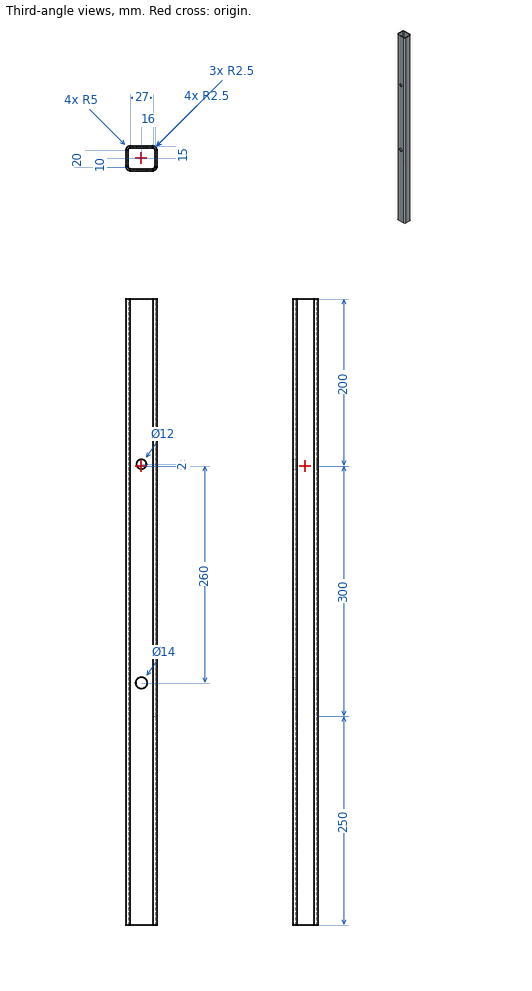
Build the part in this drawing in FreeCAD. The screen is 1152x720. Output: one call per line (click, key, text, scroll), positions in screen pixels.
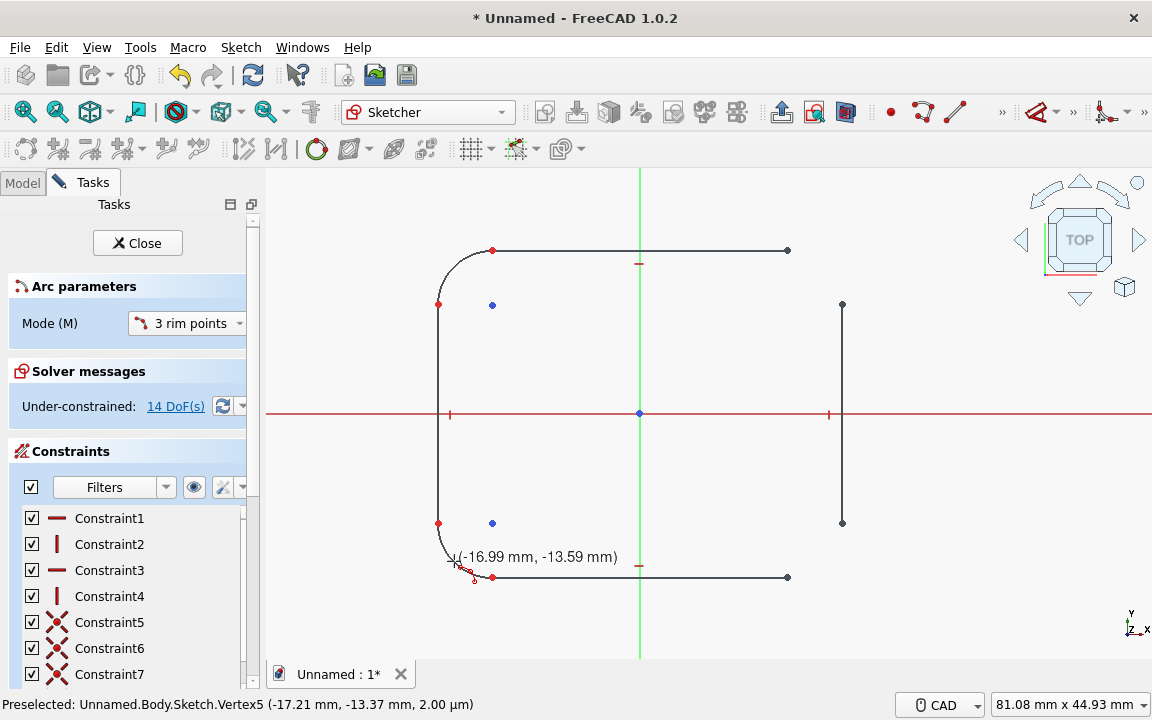
click(787, 578)
click(842, 524)
click(826, 561)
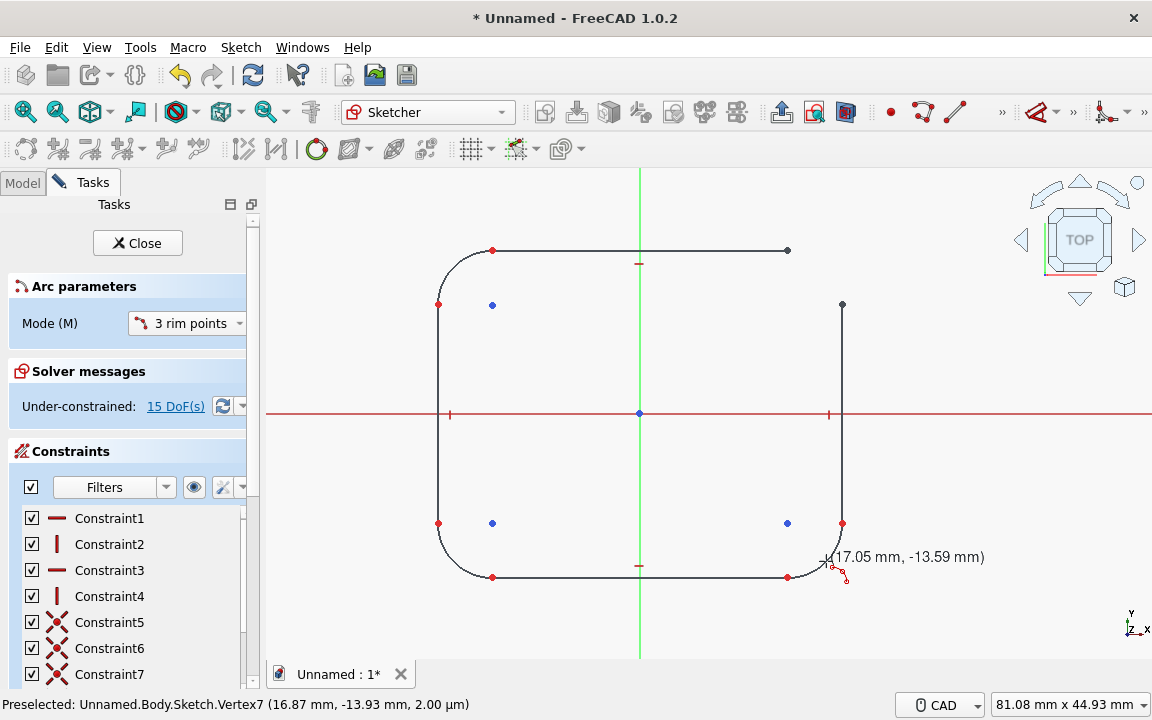
click(842, 305)
click(787, 251)
click(826, 266)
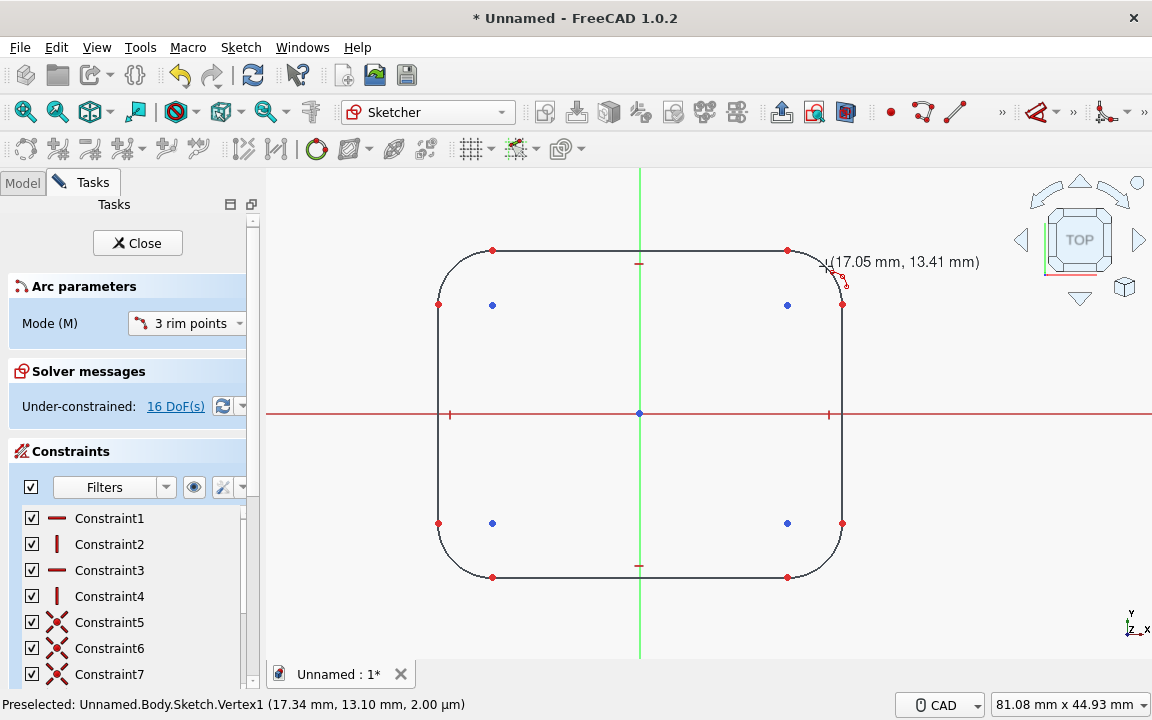
click(956, 112)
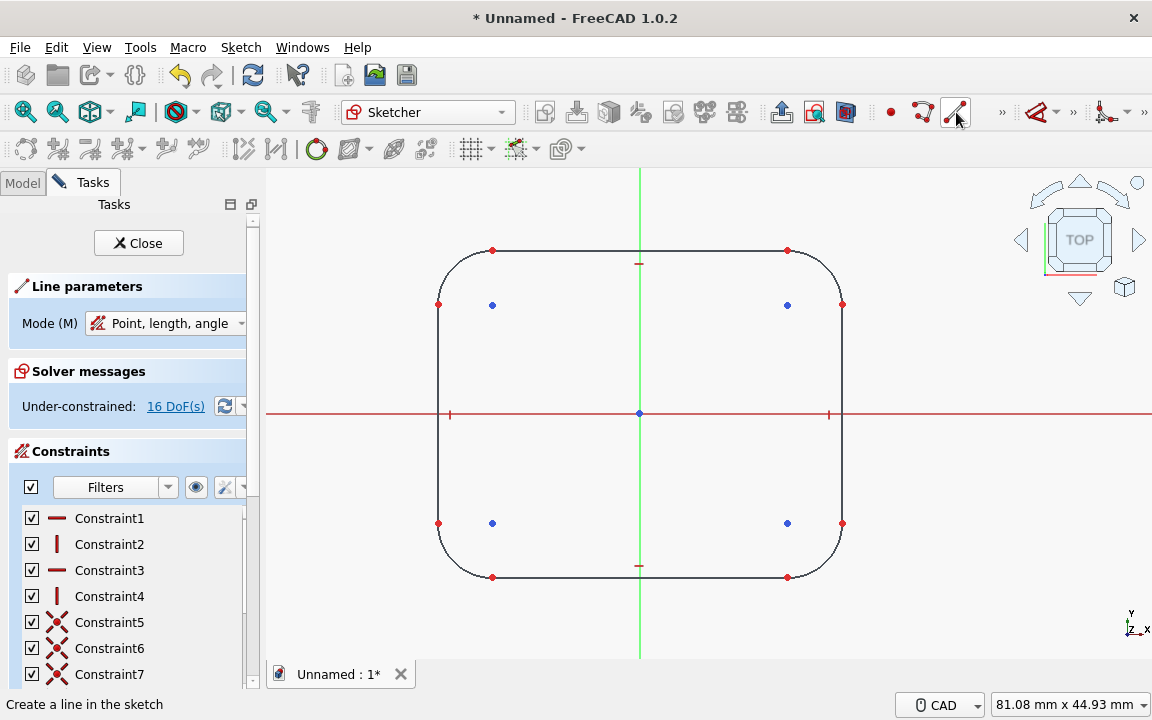
click(492, 277)
click(787, 277)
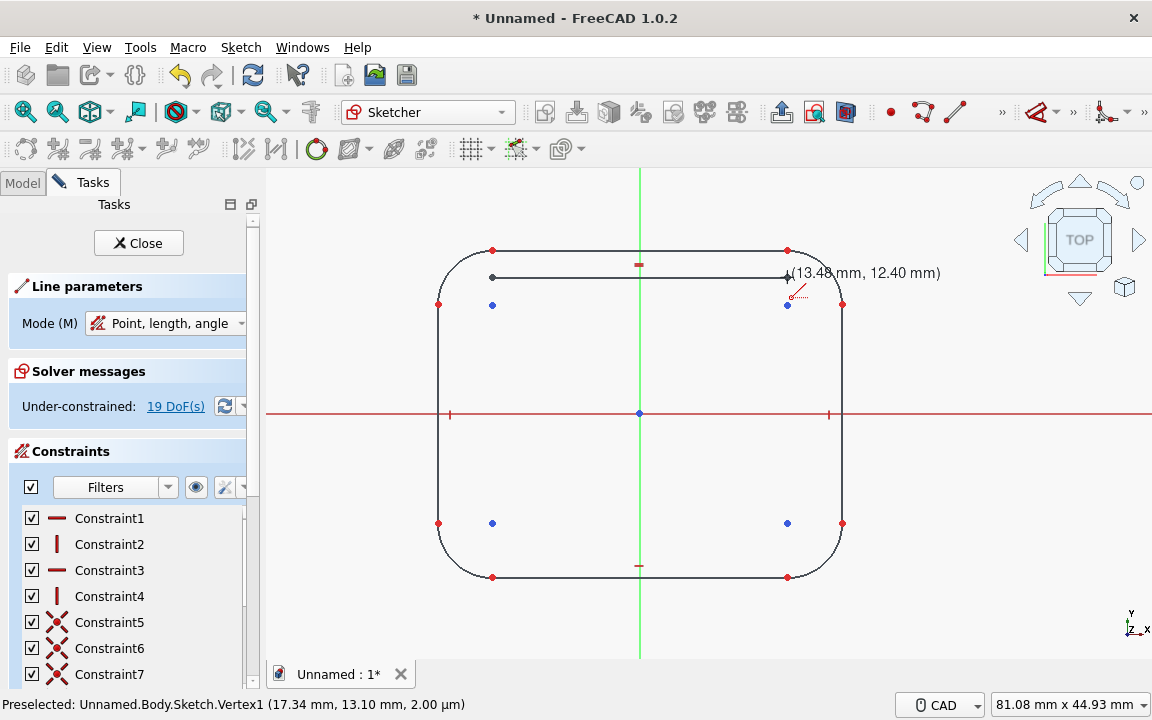
click(815, 304)
click(815, 523)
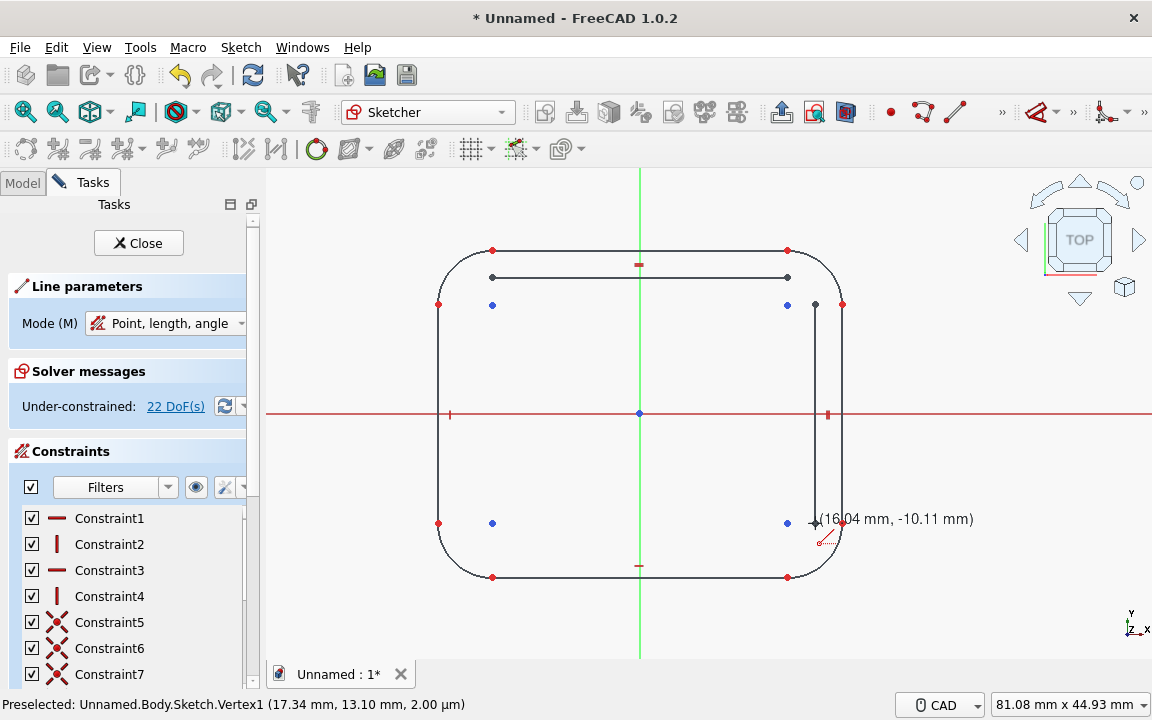
click(787, 550)
click(492, 550)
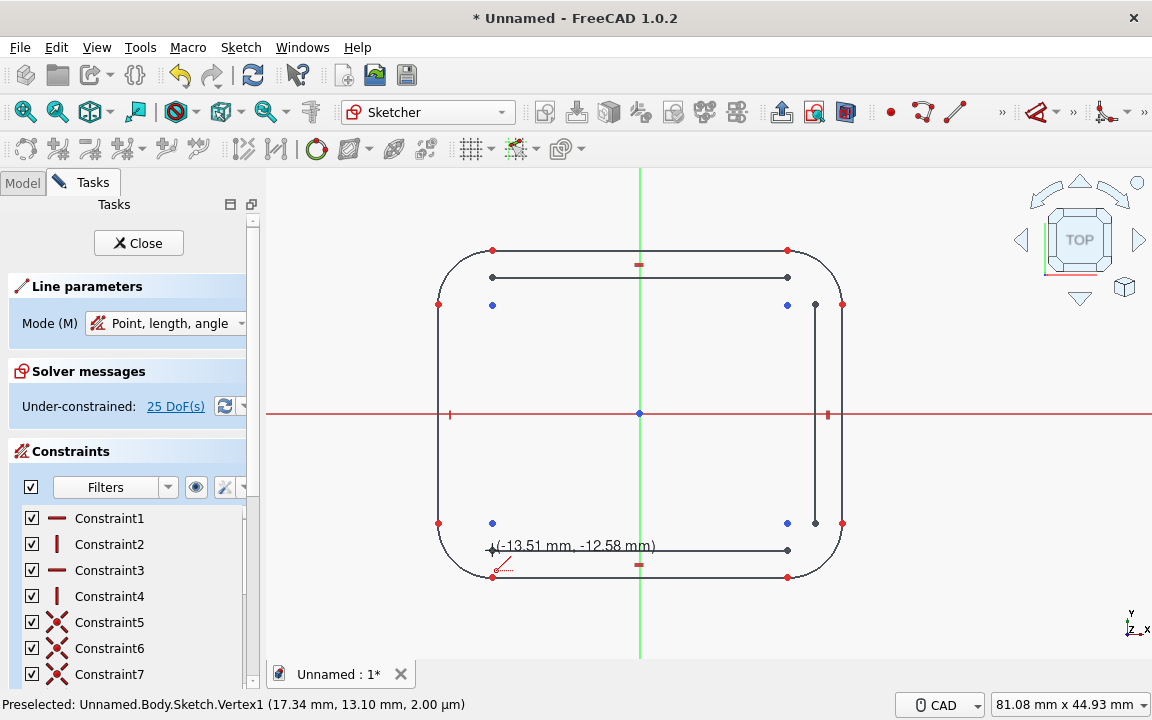
click(465, 523)
click(465, 304)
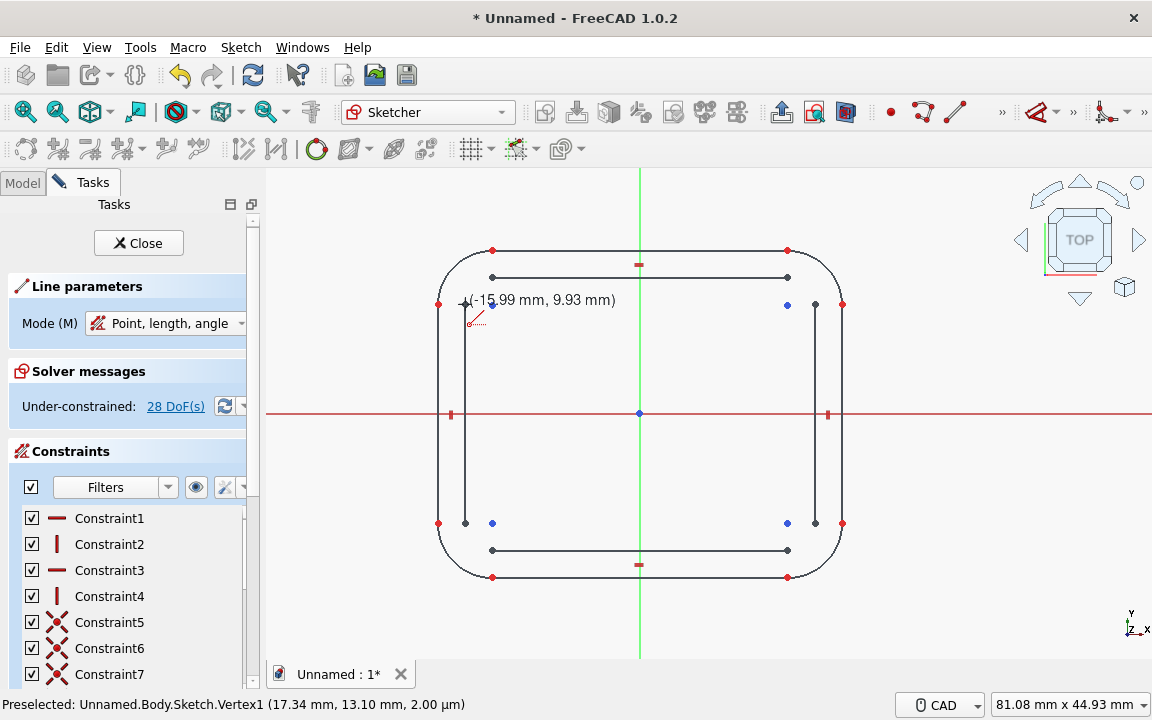
key(g)
key(3)
key(a)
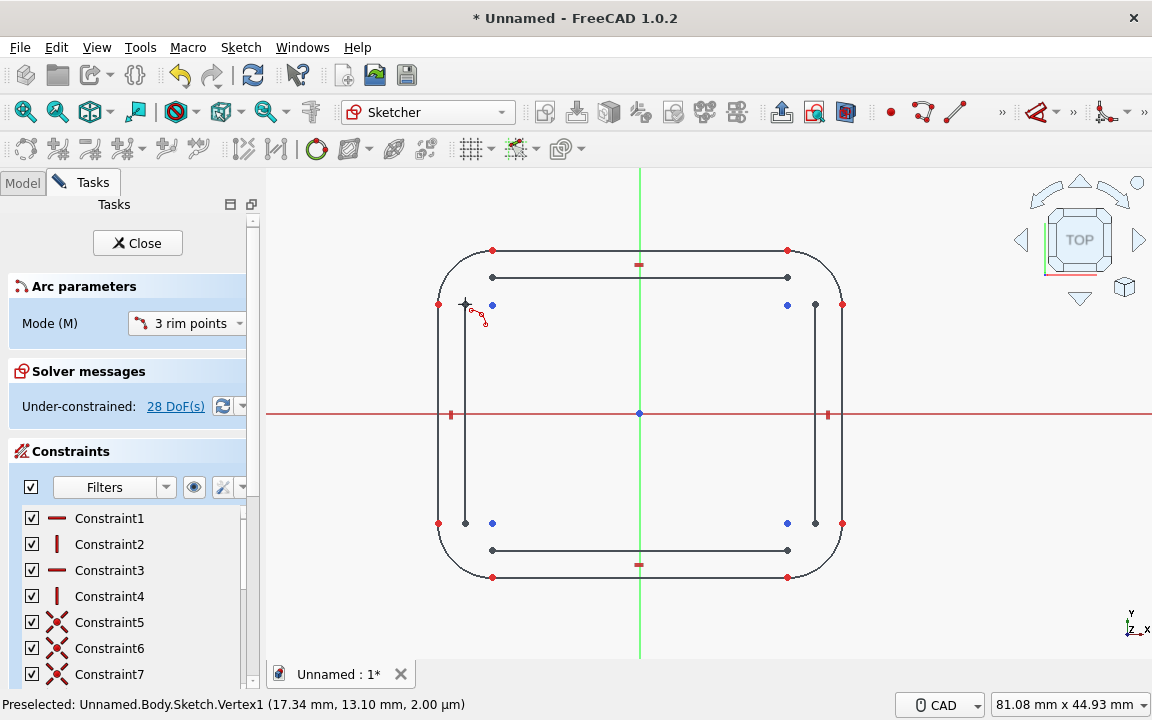
click(787, 278)
click(815, 305)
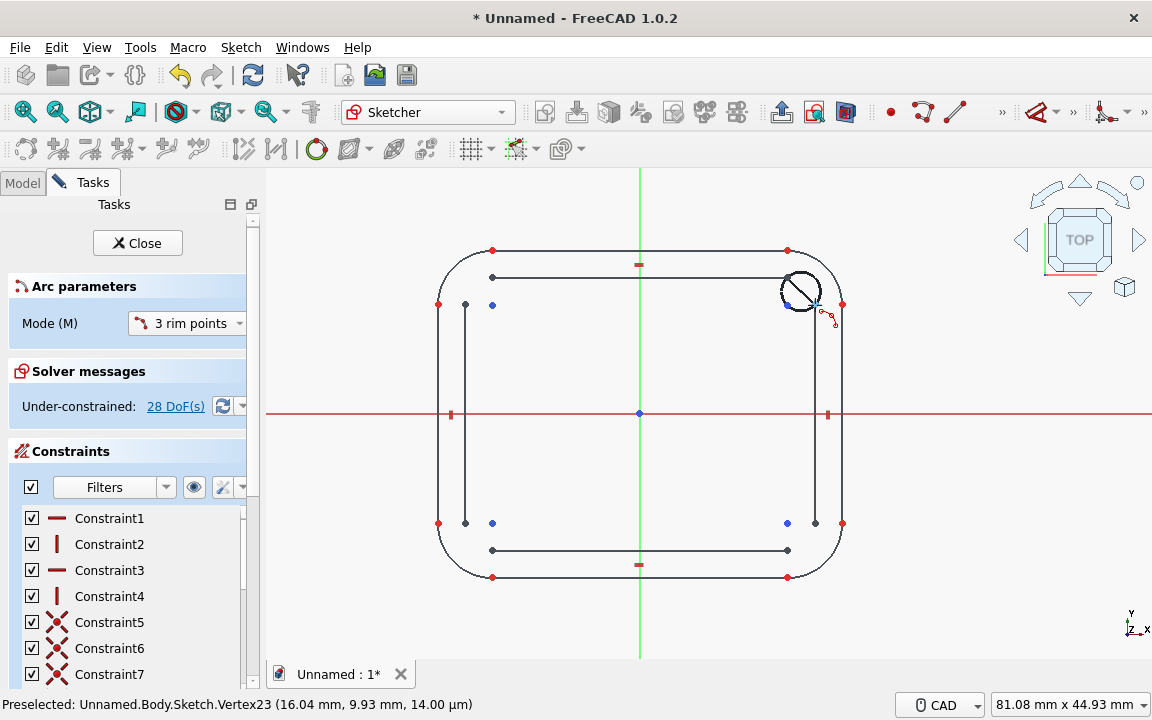
scroll(807, 285, up, 4)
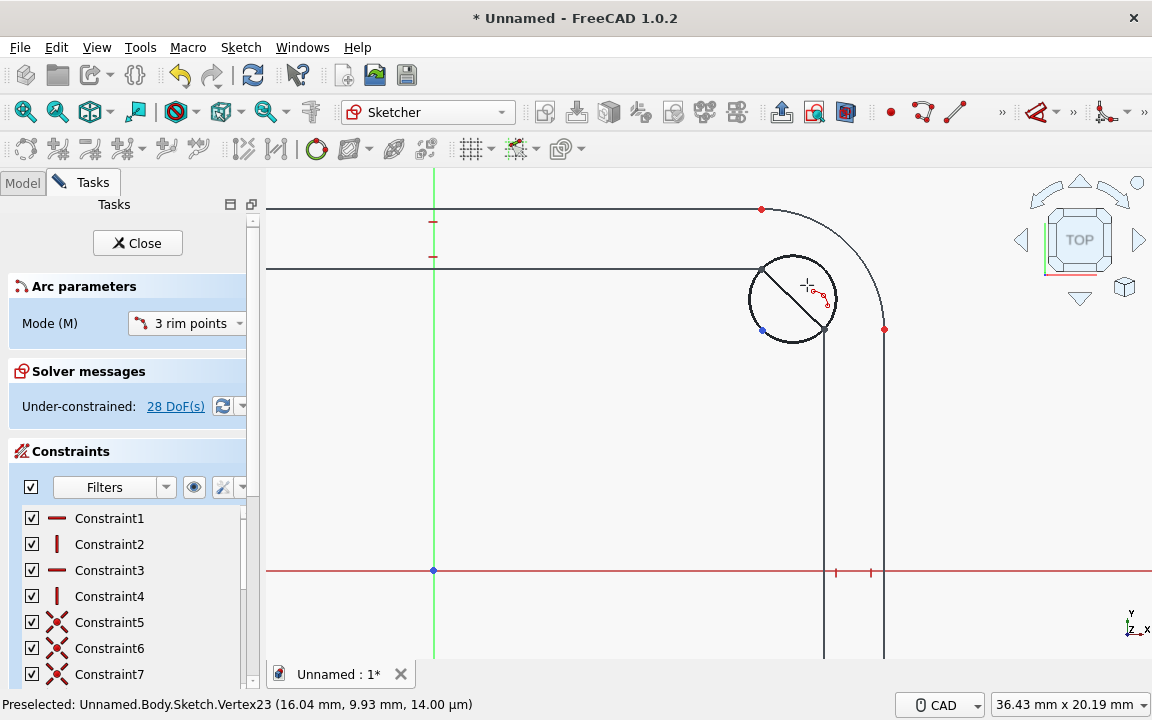
click(805, 285)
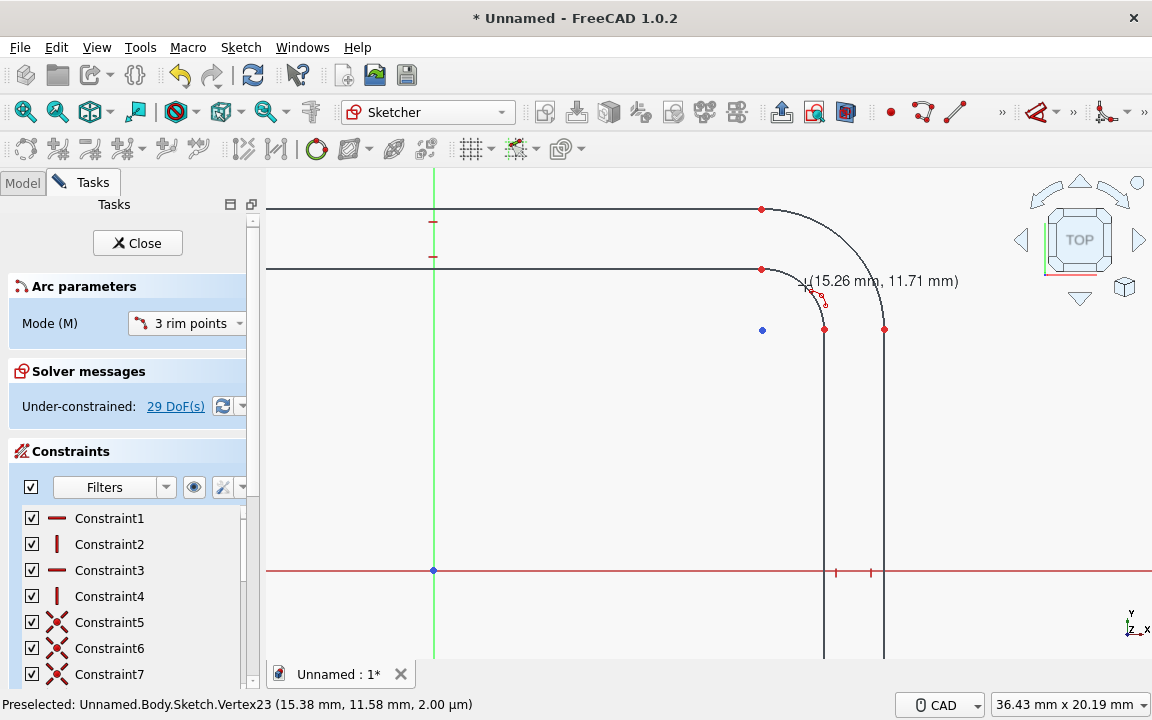
scroll(809, 285, down, 4)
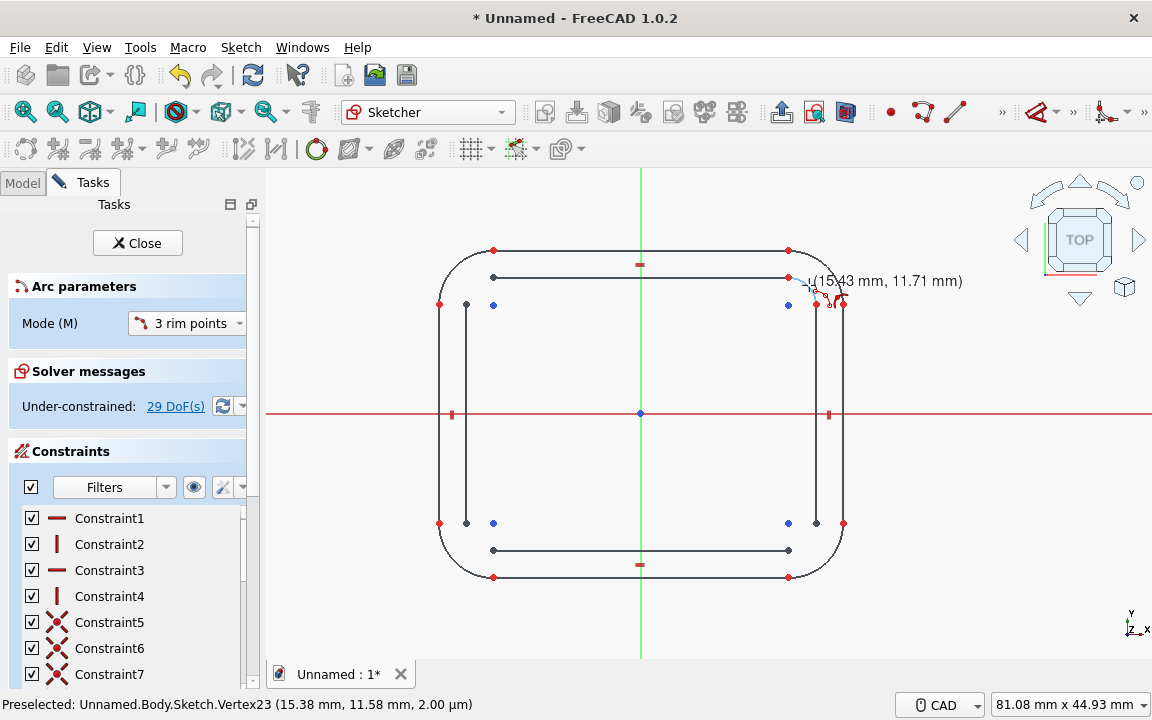
click(816, 524)
click(788, 551)